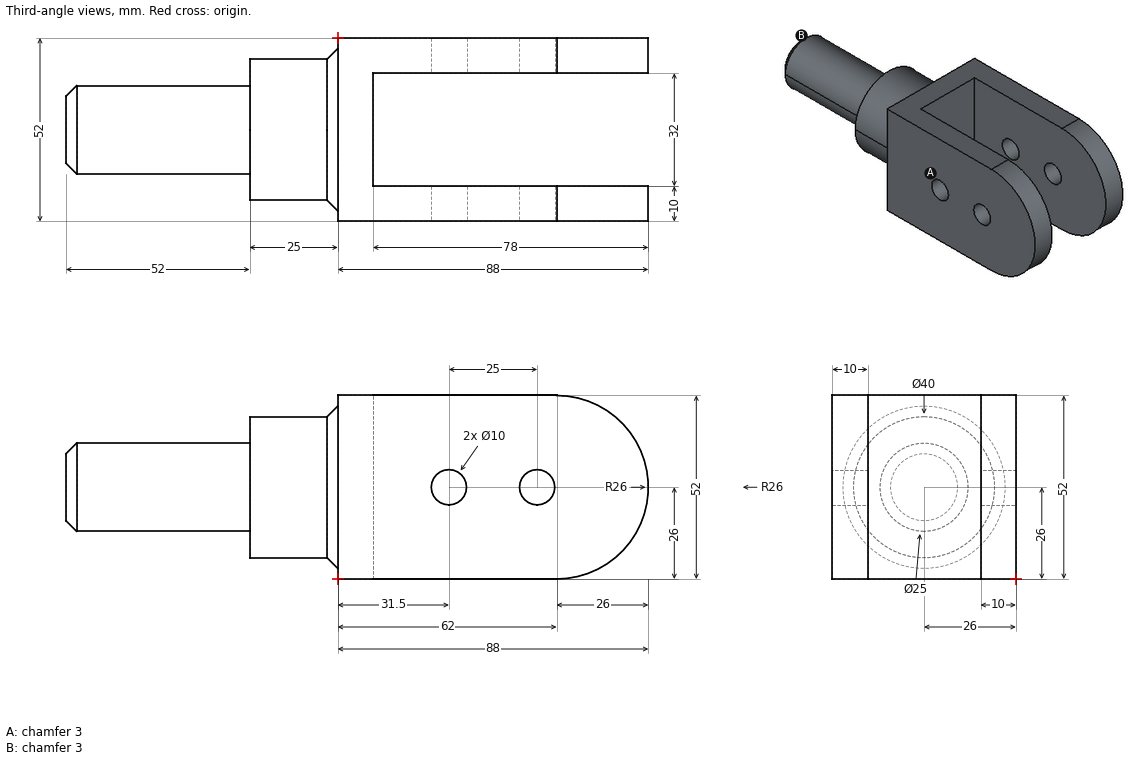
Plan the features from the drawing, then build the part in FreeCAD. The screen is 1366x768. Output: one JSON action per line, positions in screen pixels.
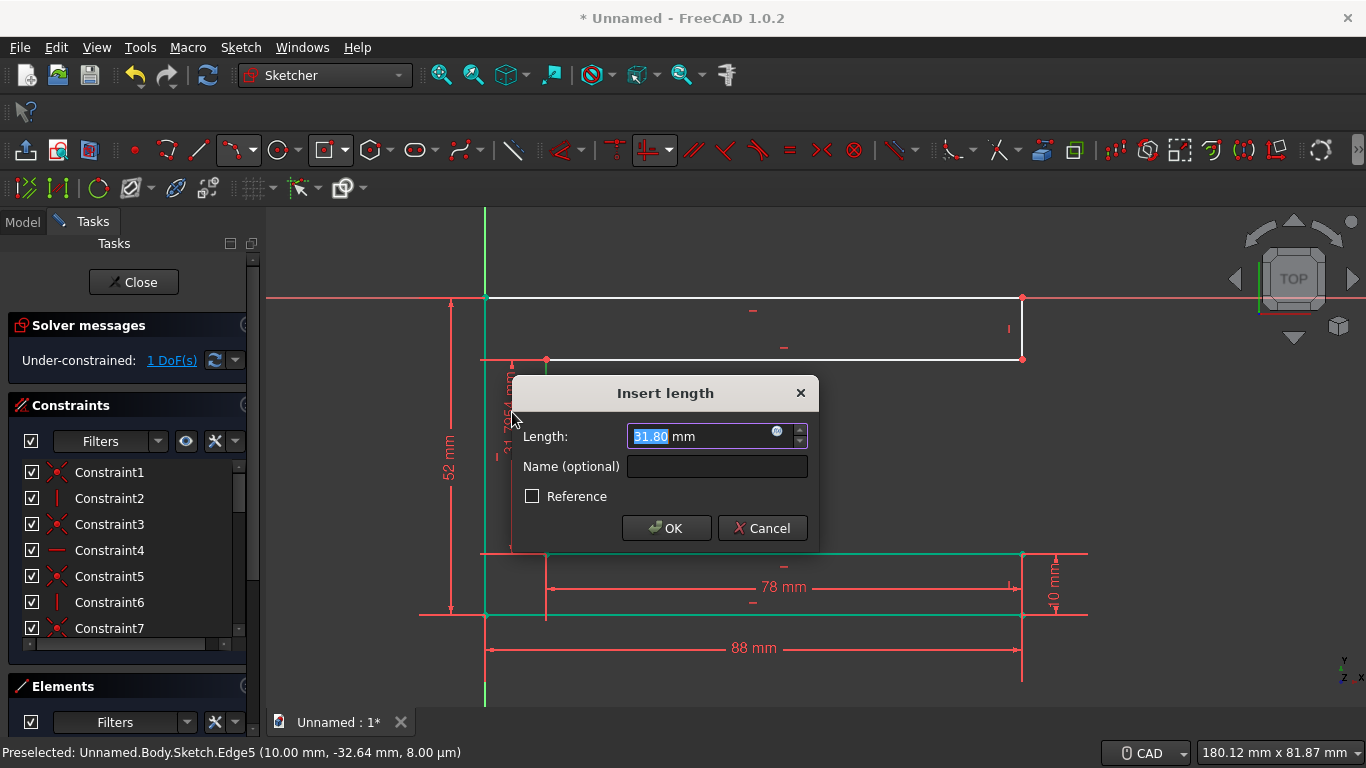
{"action": "type", "text": "32"}
{"action": "key", "text": "Return"}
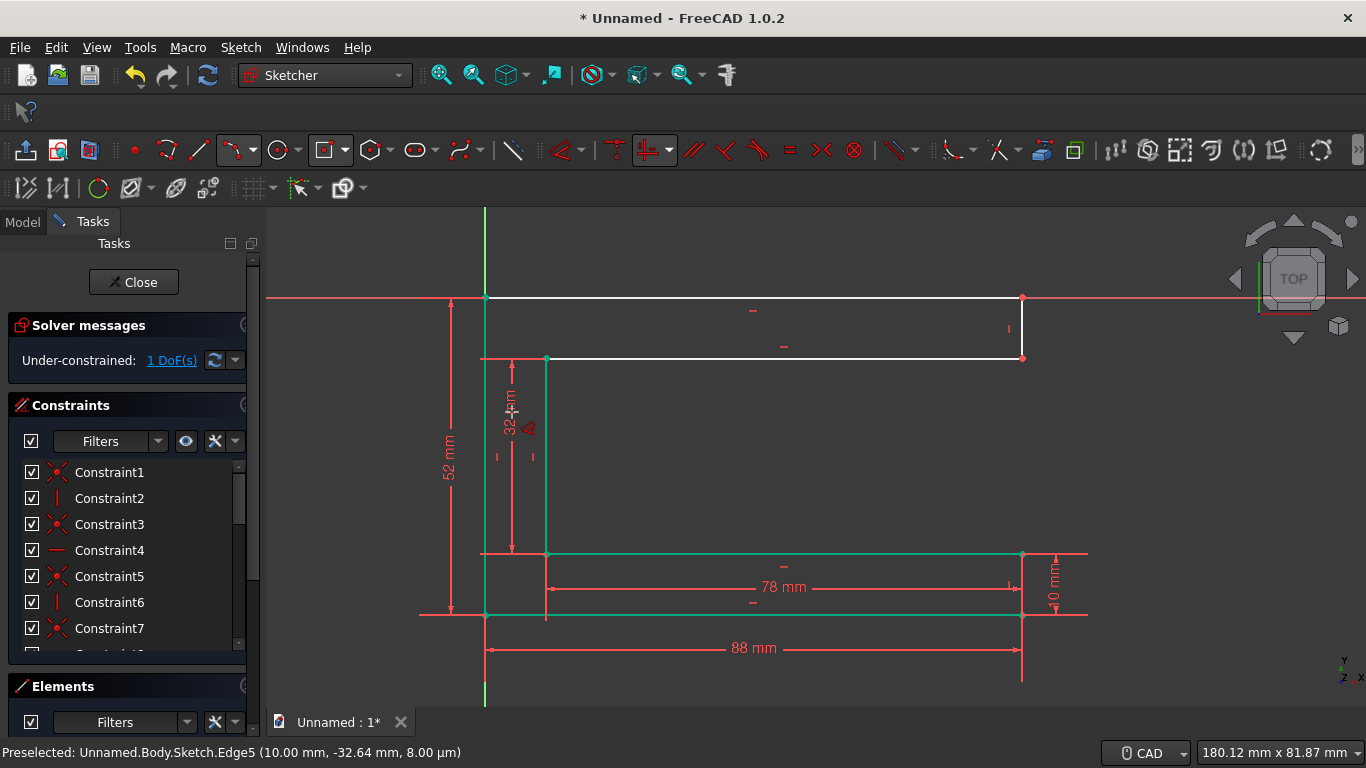
{"action": "left_click", "coordinate": [689, 359]}
{"action": "left_click", "coordinate": [784, 325]}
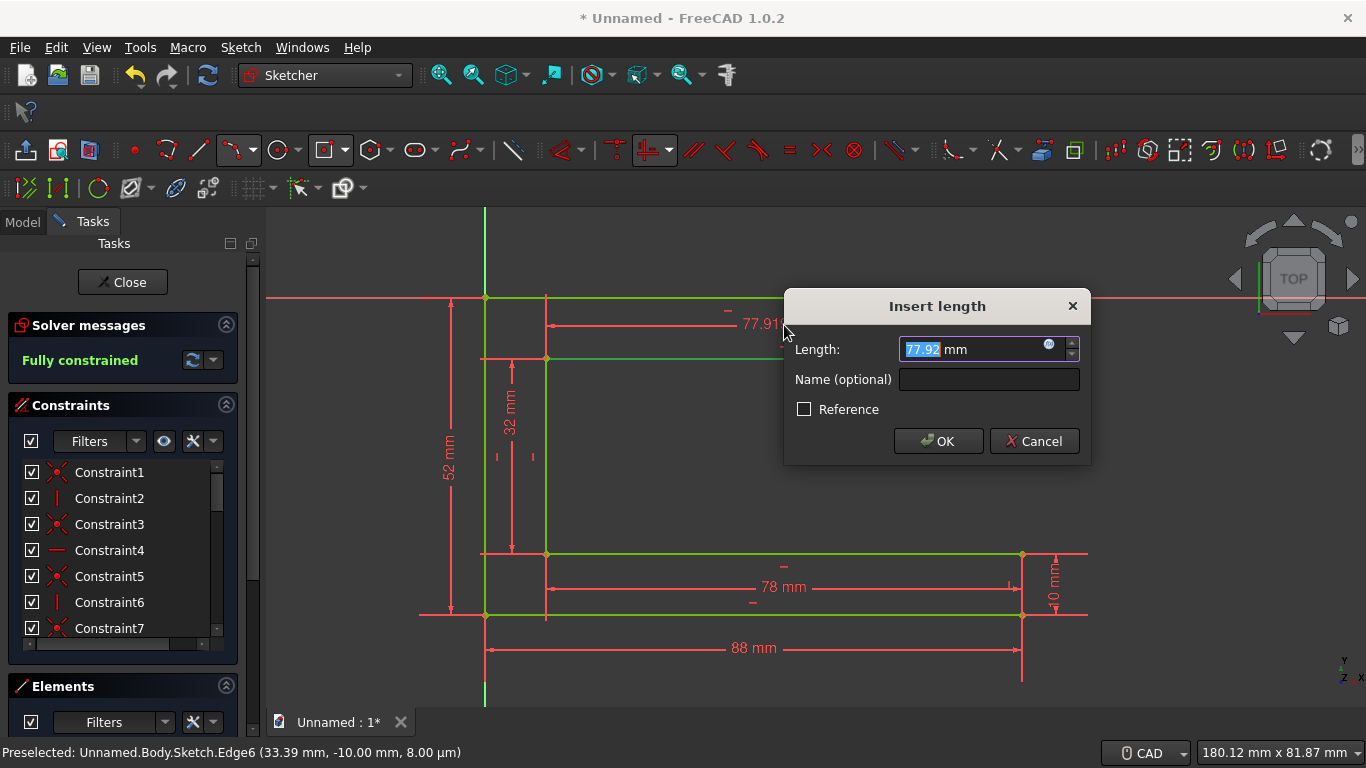
{"action": "type", "text": "78"}
{"action": "key", "text": "Return"}
{"action": "key", "text": "Escape"}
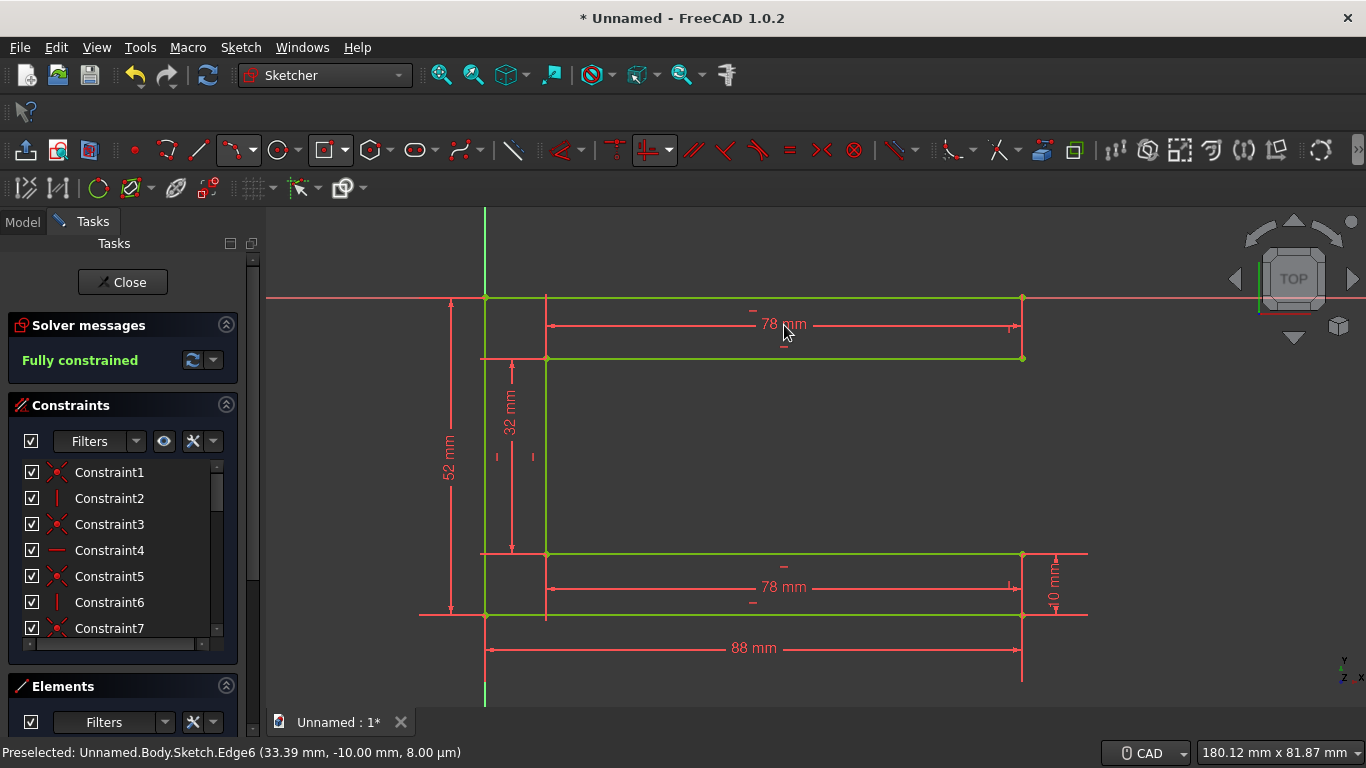
{"action": "left_click", "coordinate": [123, 282]}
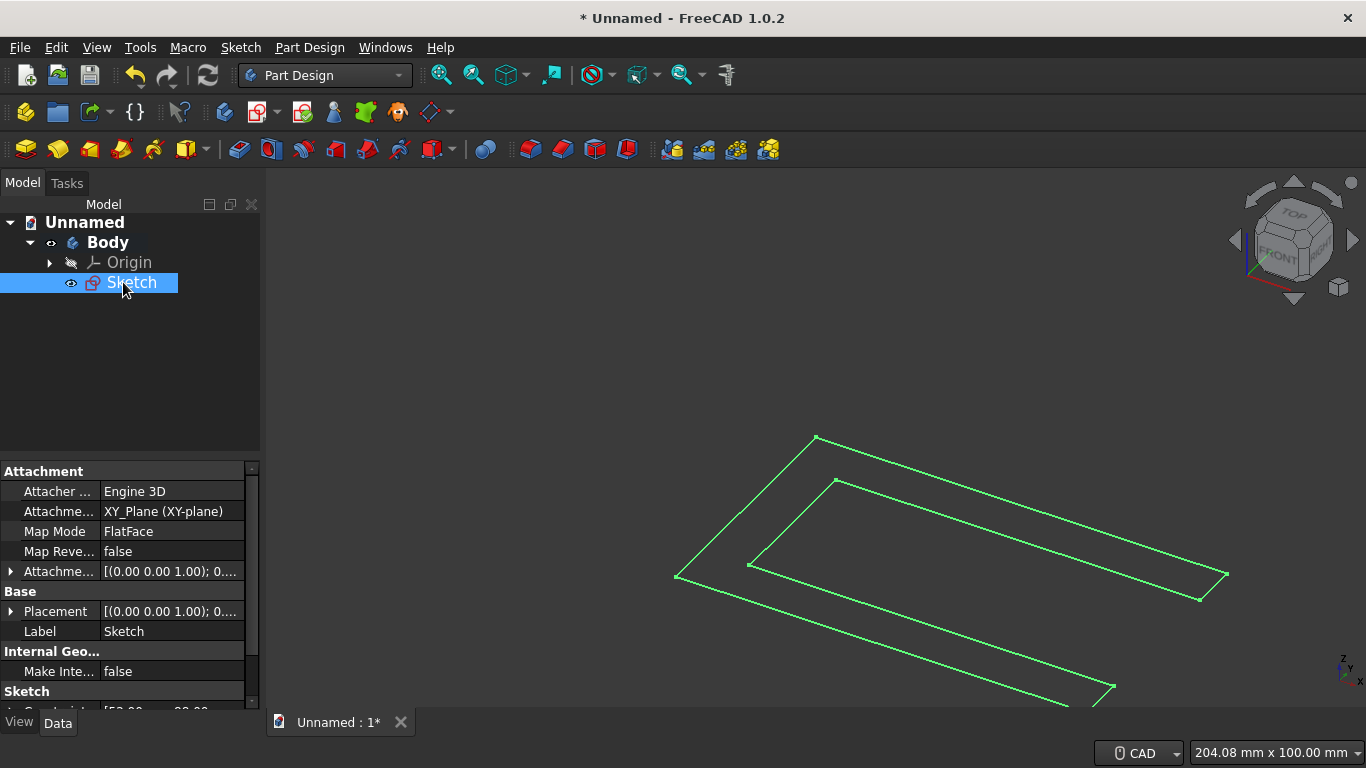
{"action": "left_click", "coordinate": [26, 150]}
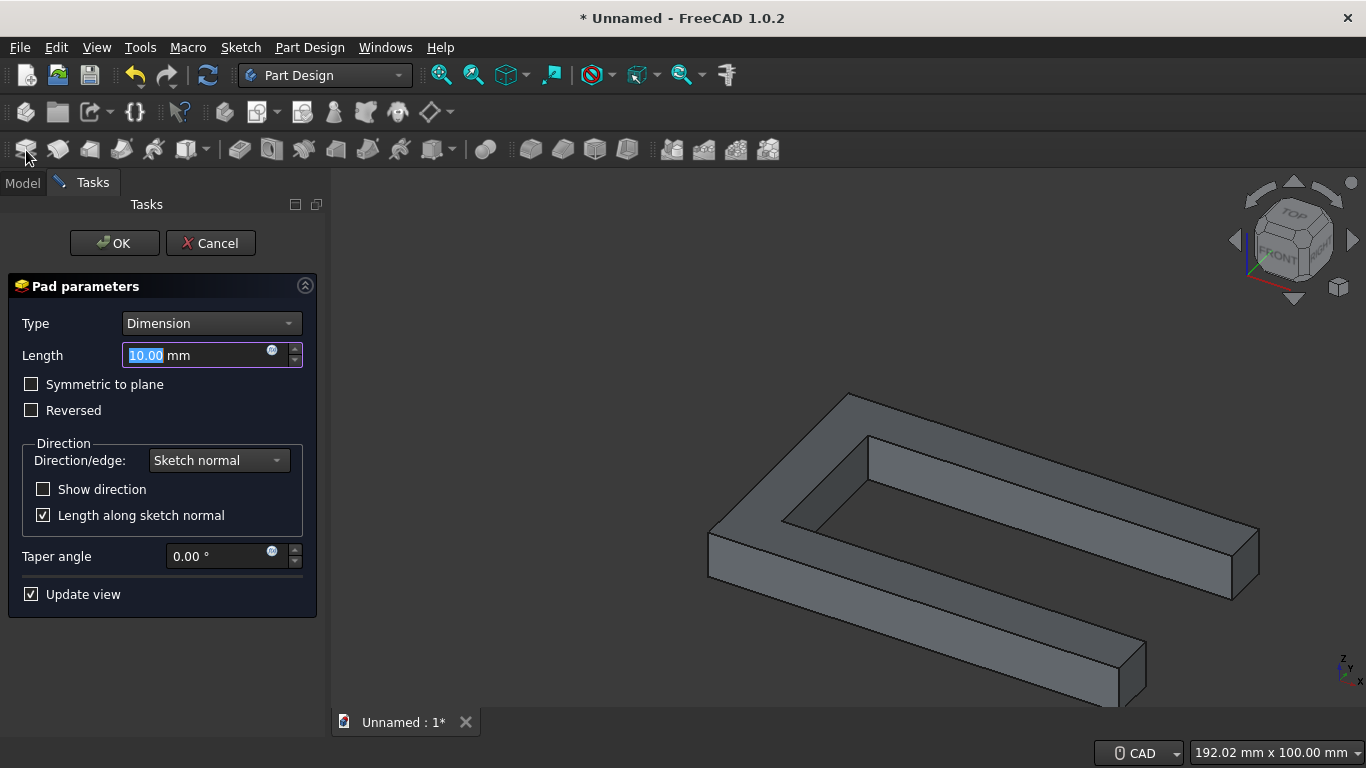
{"action": "type", "text": "52"}
{"action": "key", "text": "Tab"}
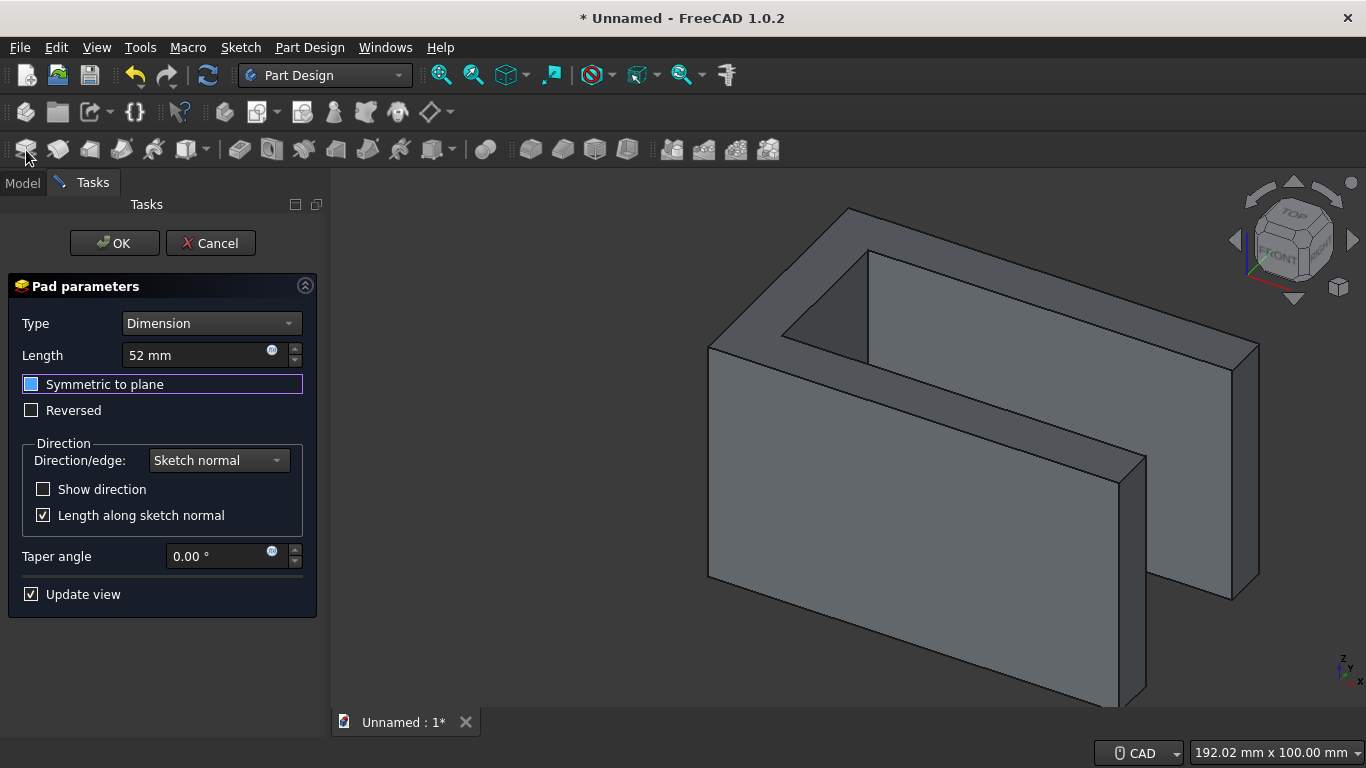
{"action": "left_click", "coordinate": [115, 243]}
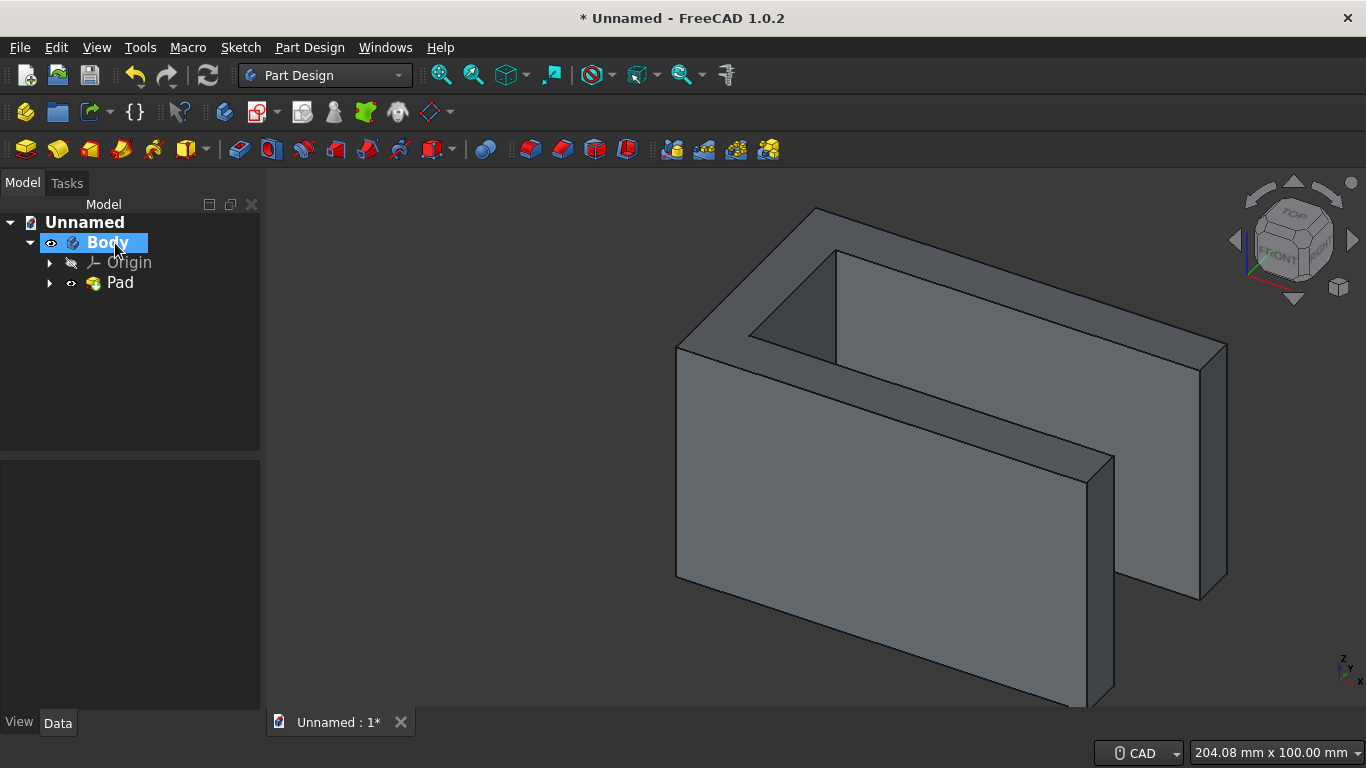
{"action": "left_click", "coordinate": [442, 76]}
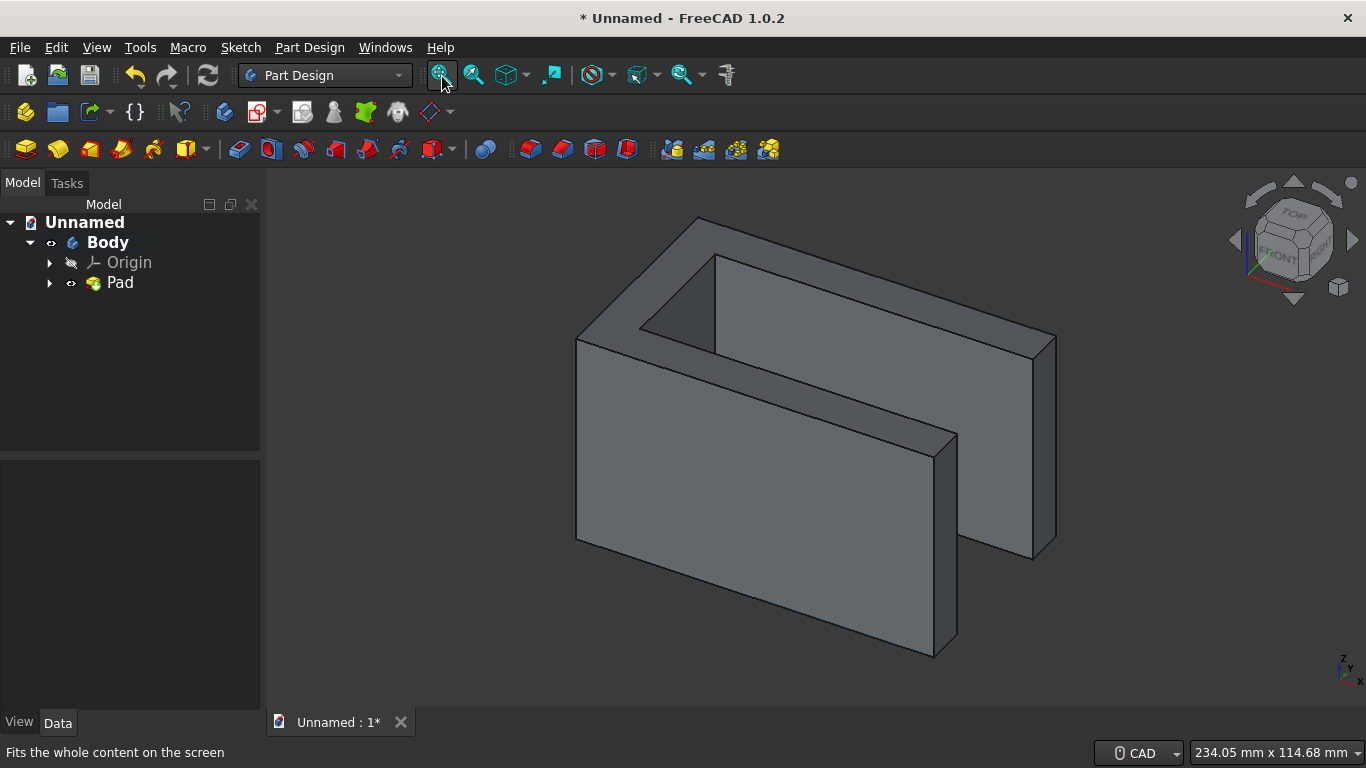
{"action": "left_click", "coordinate": [258, 112]}